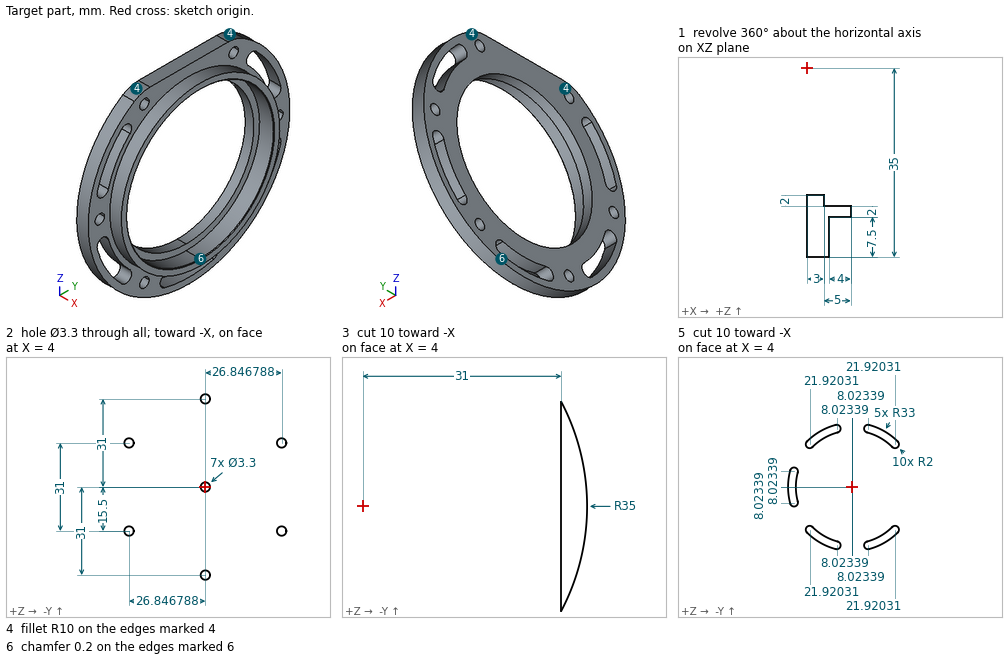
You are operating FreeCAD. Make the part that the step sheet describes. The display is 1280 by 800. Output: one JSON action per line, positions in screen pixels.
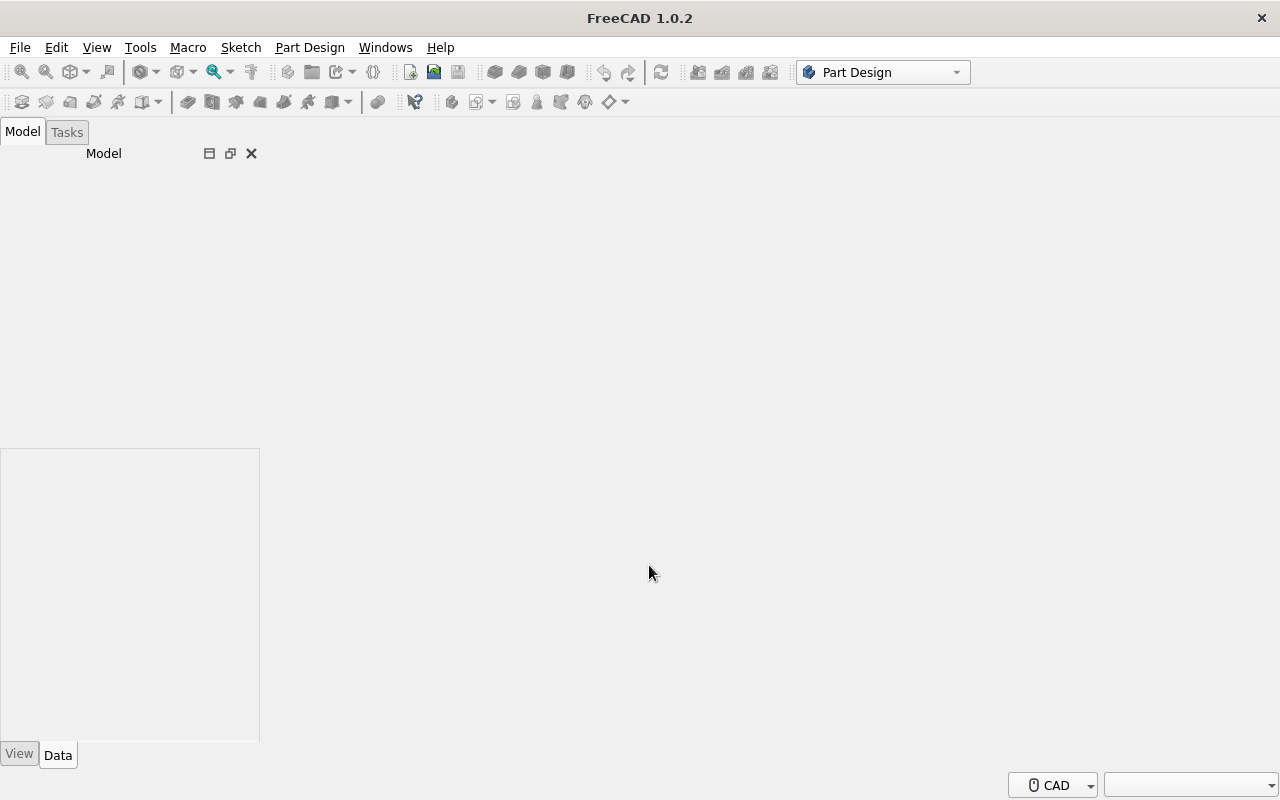
{"action": "left_click", "coordinate": [410, 72]}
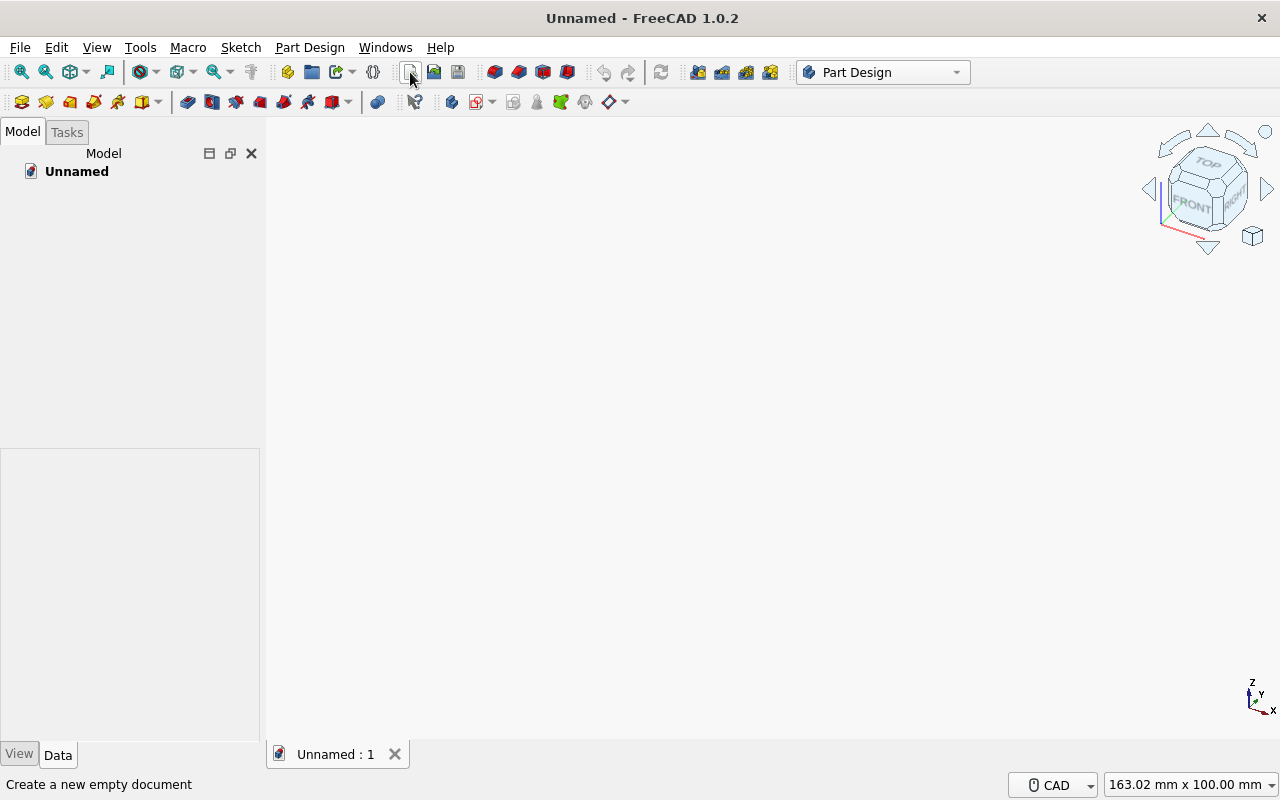
{"action": "left_click", "coordinate": [476, 102]}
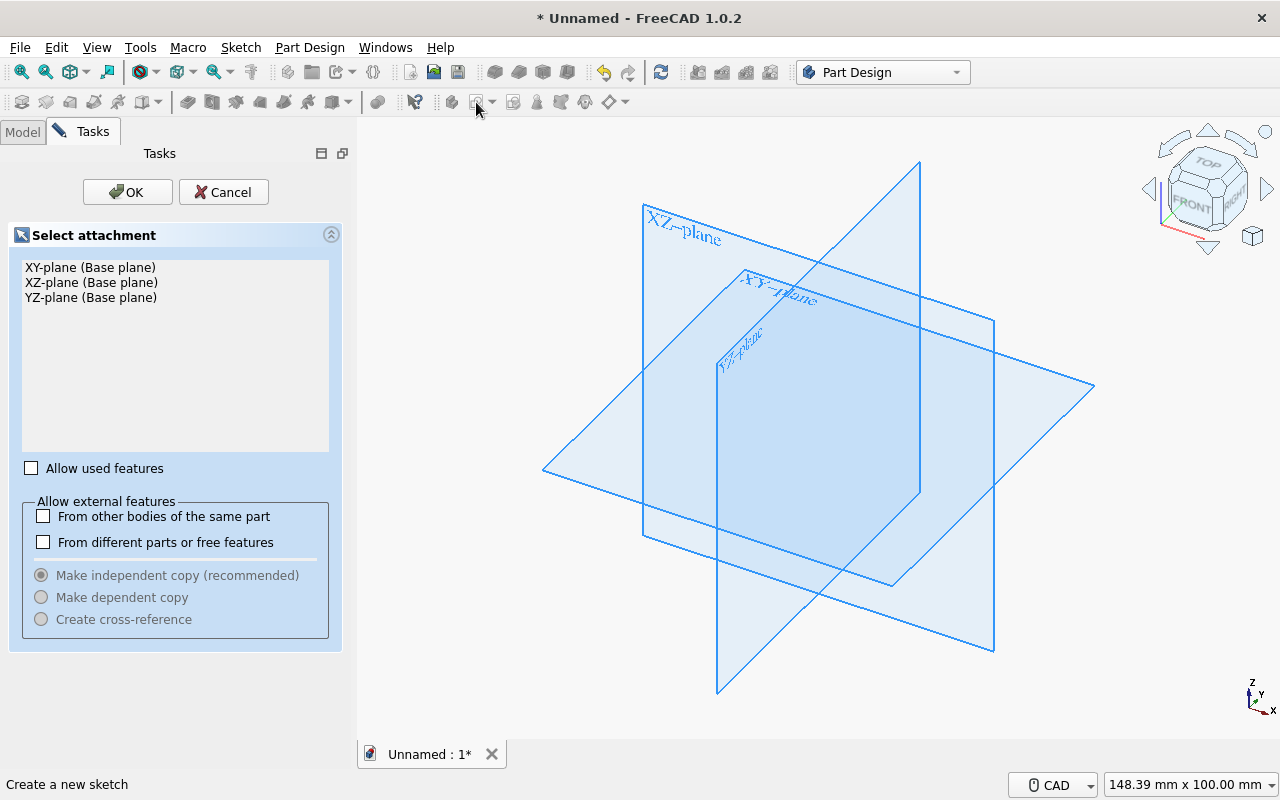
{"action": "left_click", "coordinate": [82, 282]}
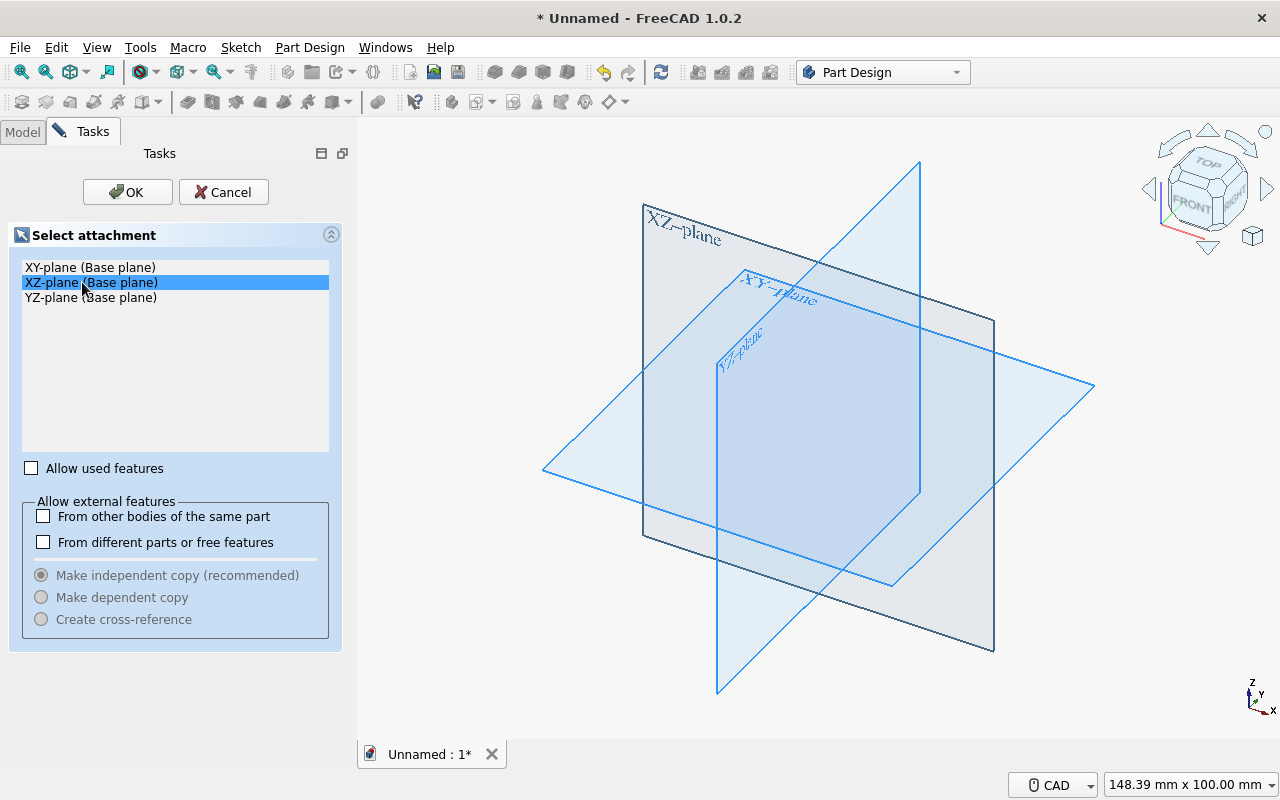
{"action": "left_click", "coordinate": [128, 192]}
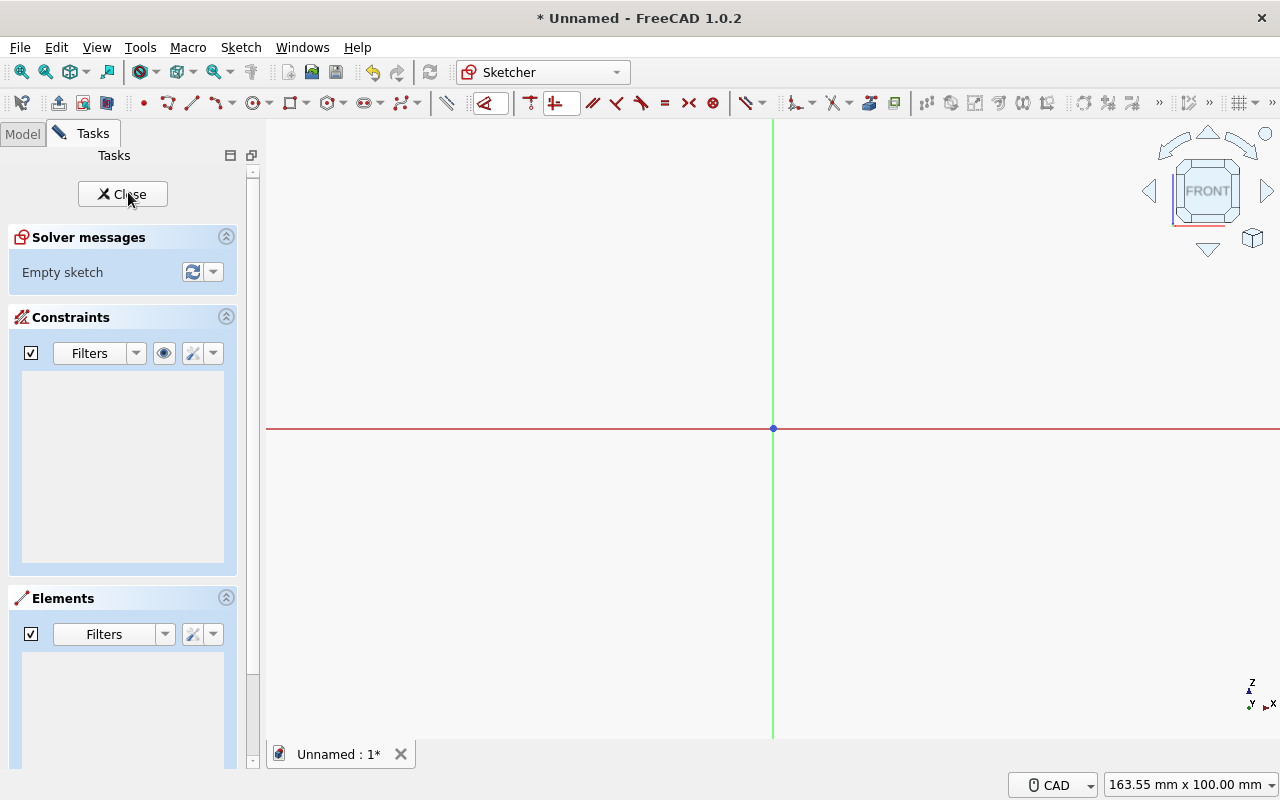
{"action": "scroll", "coordinate": [816, 646], "scroll_direction": "up", "scroll_amount": 9}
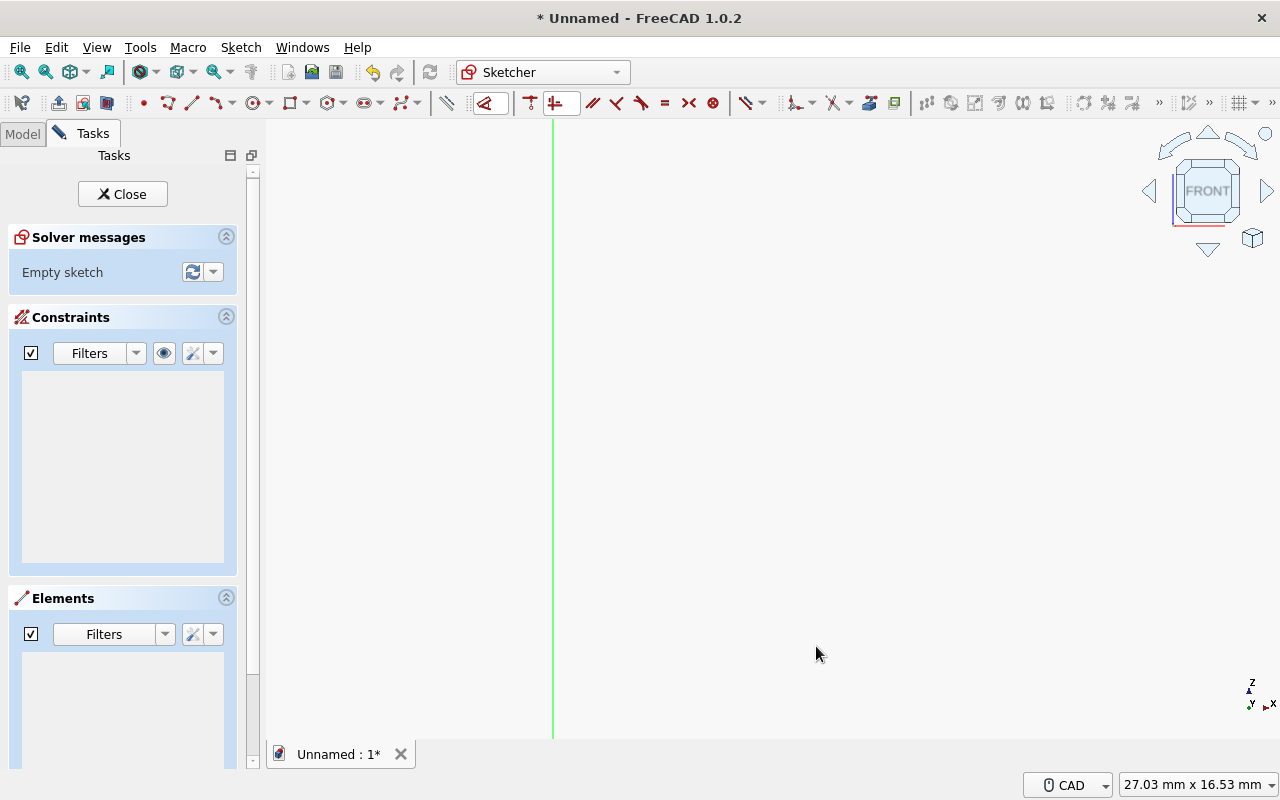
{"action": "left_click", "coordinate": [168, 104]}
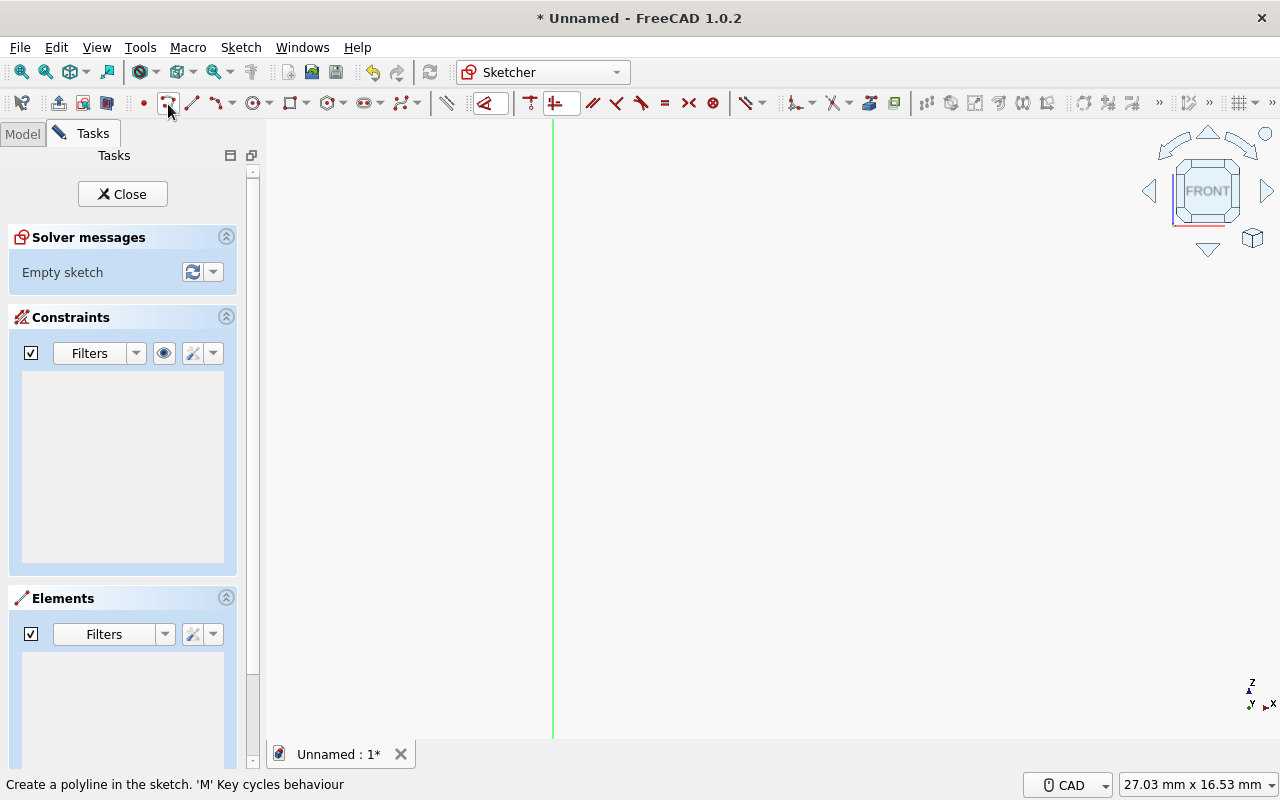
{"action": "left_click", "coordinate": [553, 210]}
{"action": "left_click", "coordinate": [666, 210]}
{"action": "left_click", "coordinate": [666, 285]}
{"action": "left_click", "coordinate": [853, 285]}
{"action": "left_click", "coordinate": [853, 360]}
{"action": "left_click", "coordinate": [703, 360]}
{"action": "left_click", "coordinate": [703, 642]}
{"action": "left_click", "coordinate": [562, 642]}
{"action": "left_click", "coordinate": [553, 211]}
{"action": "key", "text": "Escape"}
{"action": "key", "text": "Escape"}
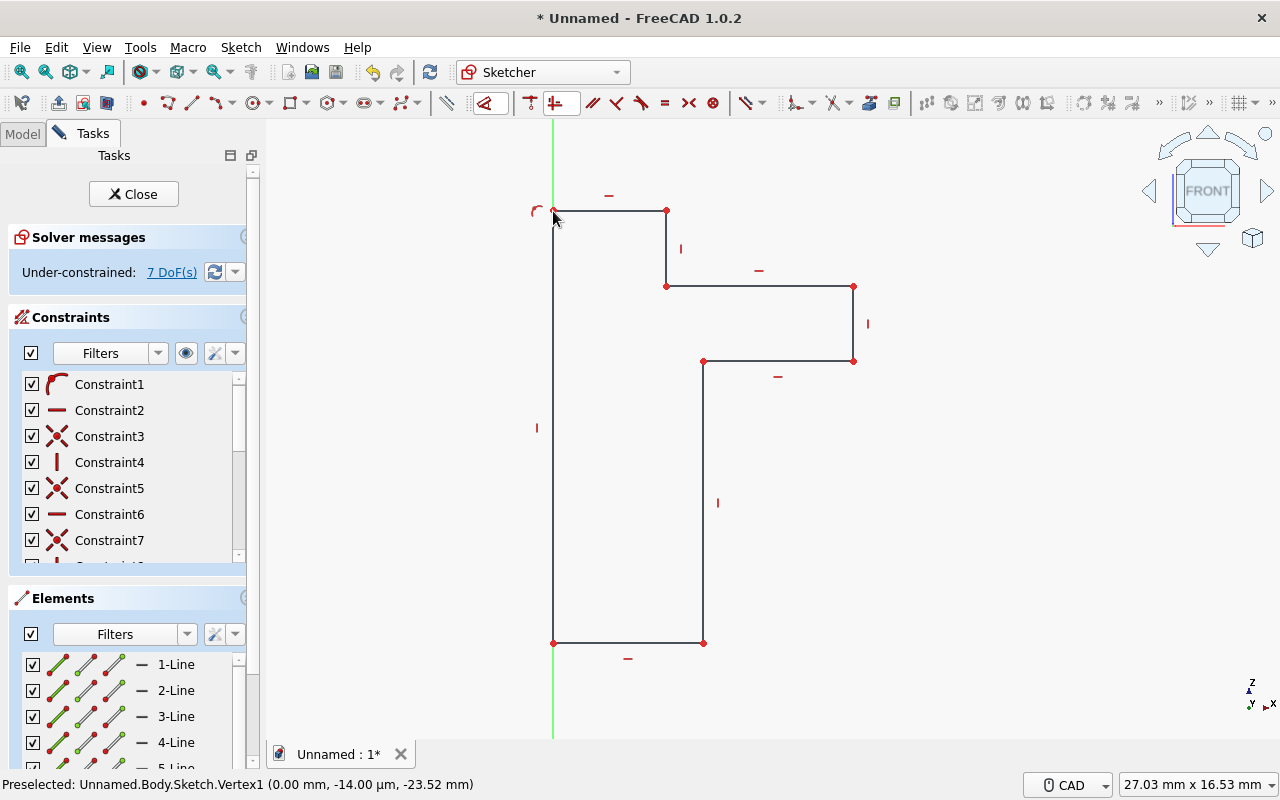
{"action": "left_click", "coordinate": [484, 104]}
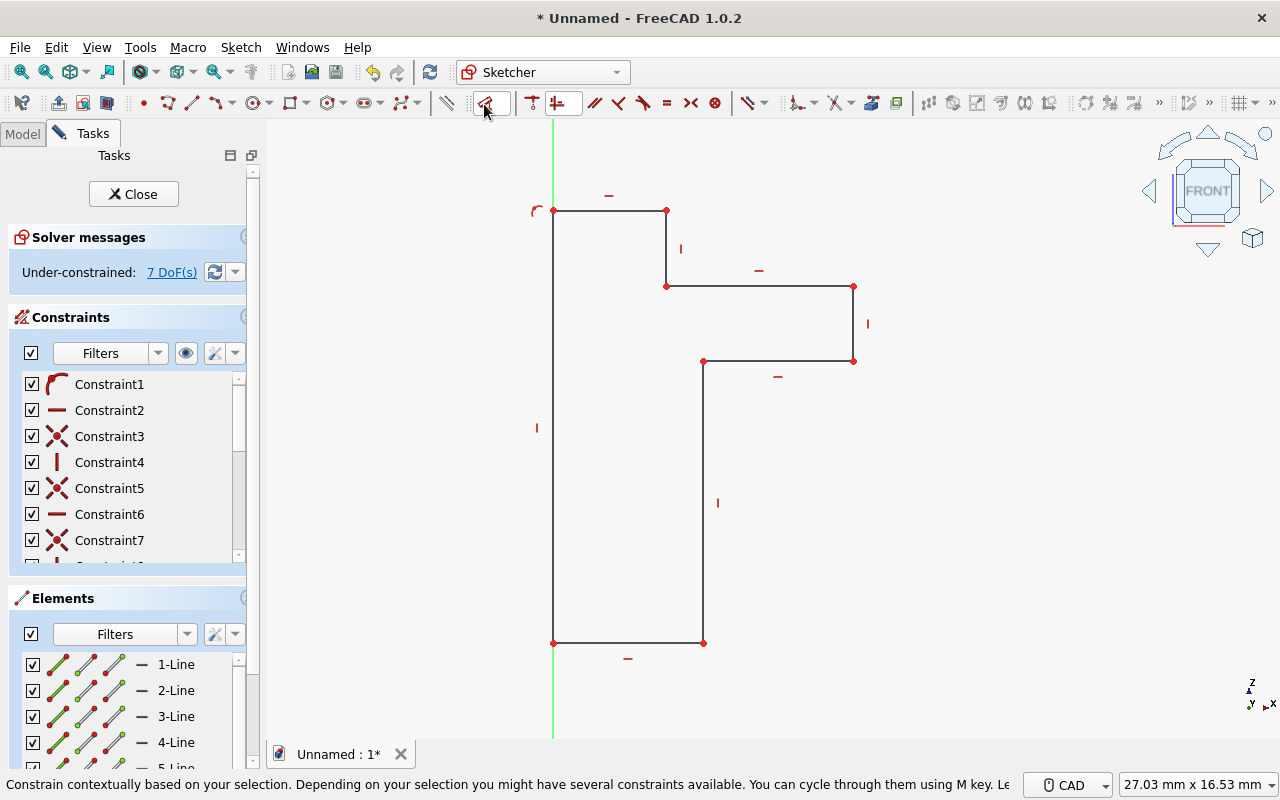
{"action": "left_click", "coordinate": [587, 211]}
{"action": "left_click", "coordinate": [610, 177]}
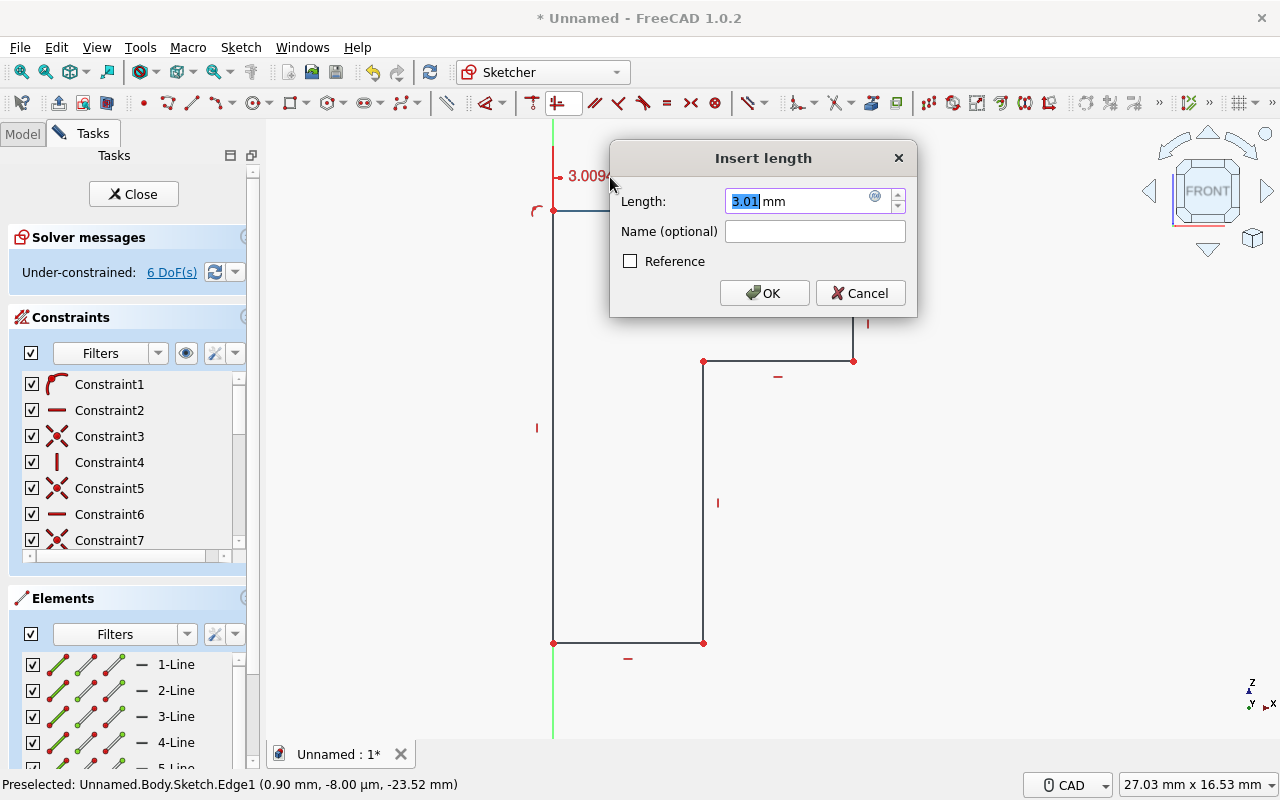
{"action": "type", "text": "3"}
{"action": "key", "text": "Return"}